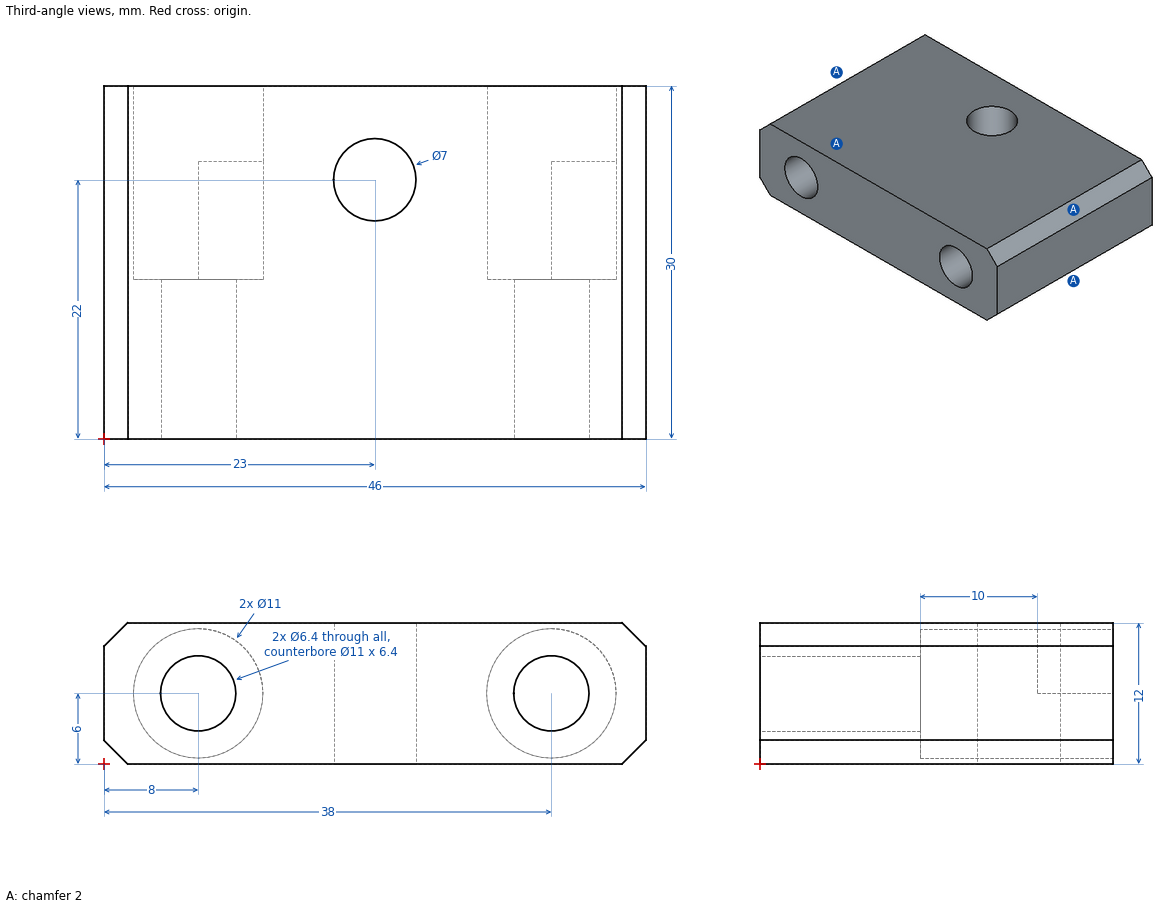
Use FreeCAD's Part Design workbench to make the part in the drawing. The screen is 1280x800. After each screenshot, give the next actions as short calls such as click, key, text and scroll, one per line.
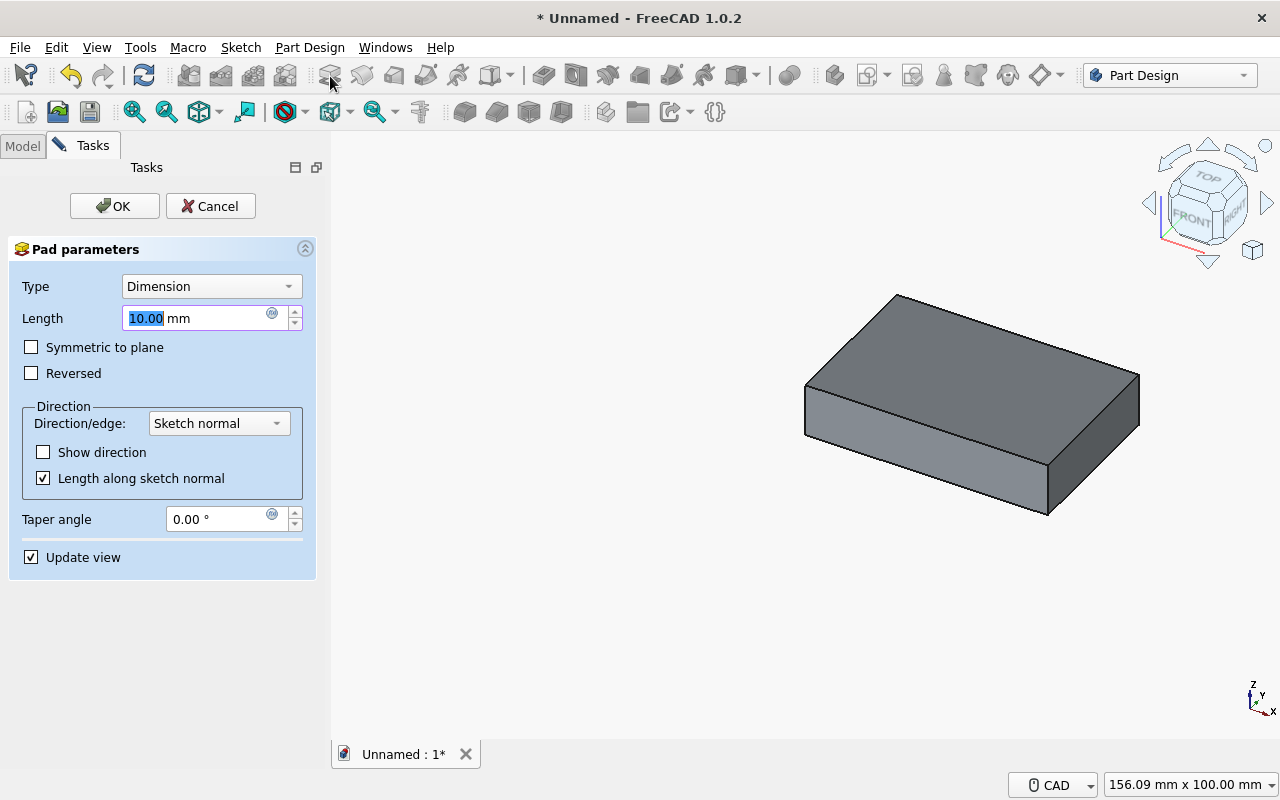
text(12)
key(Tab)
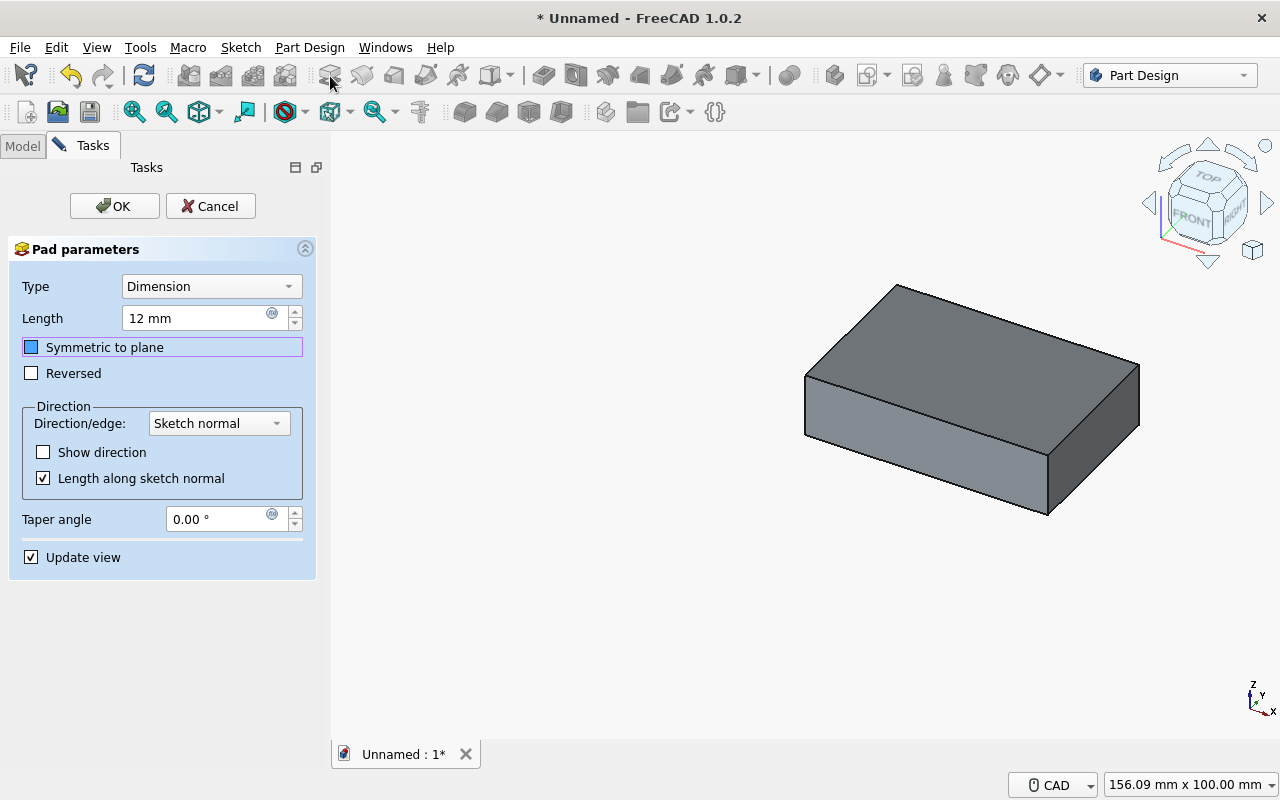
click(115, 206)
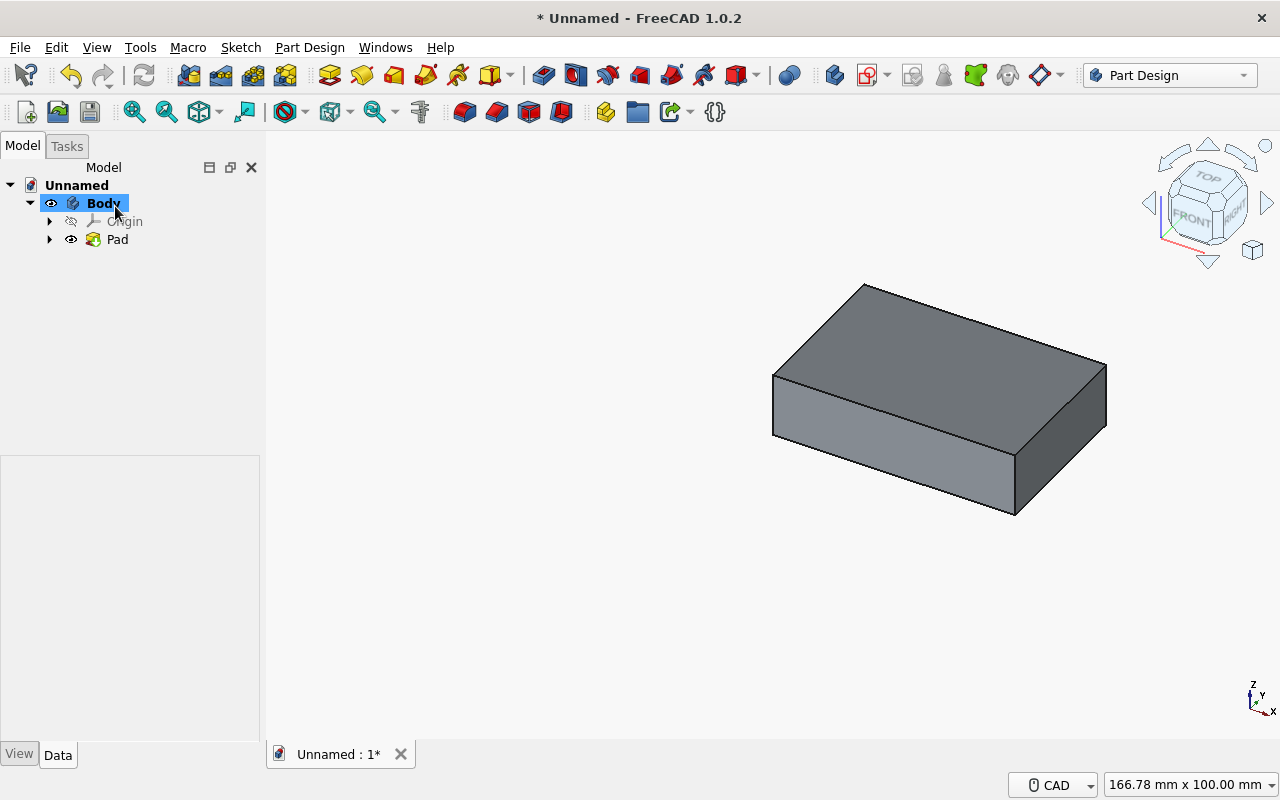
click(136, 112)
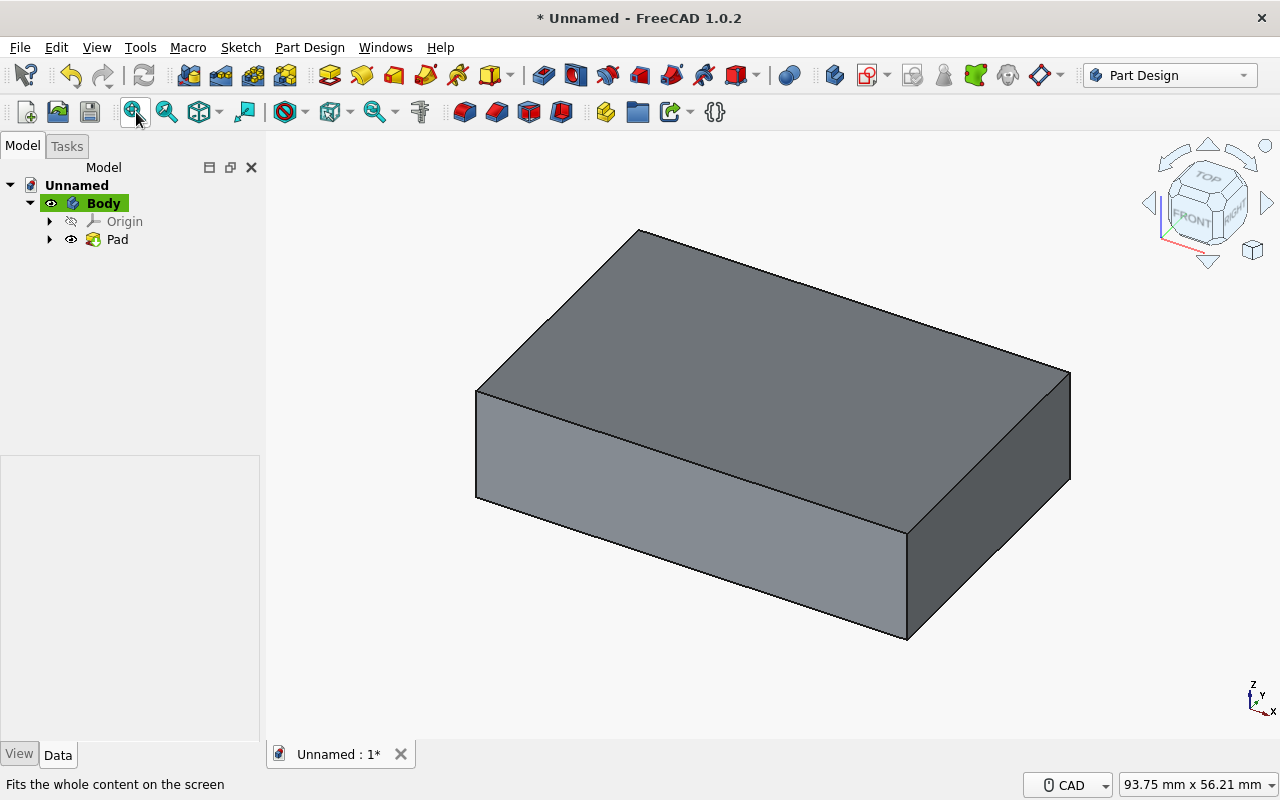
click(835, 401)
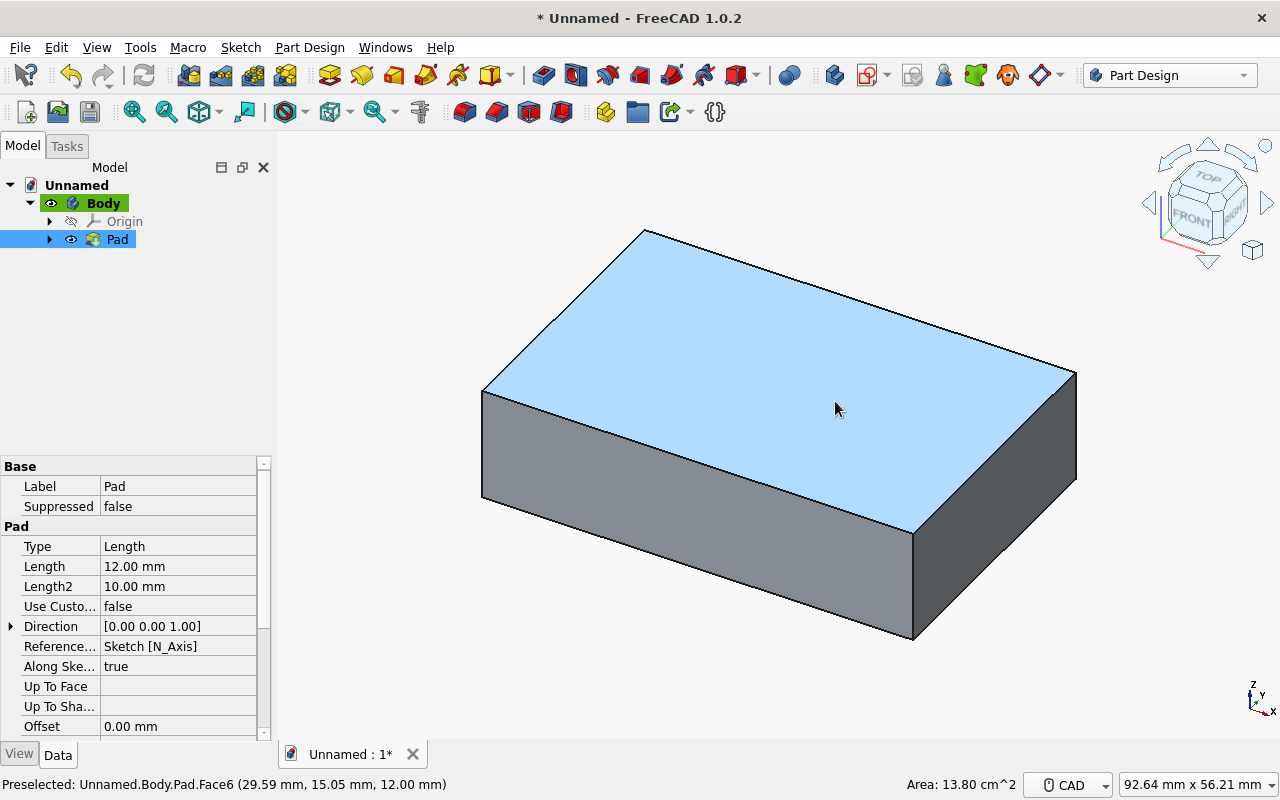
click(868, 76)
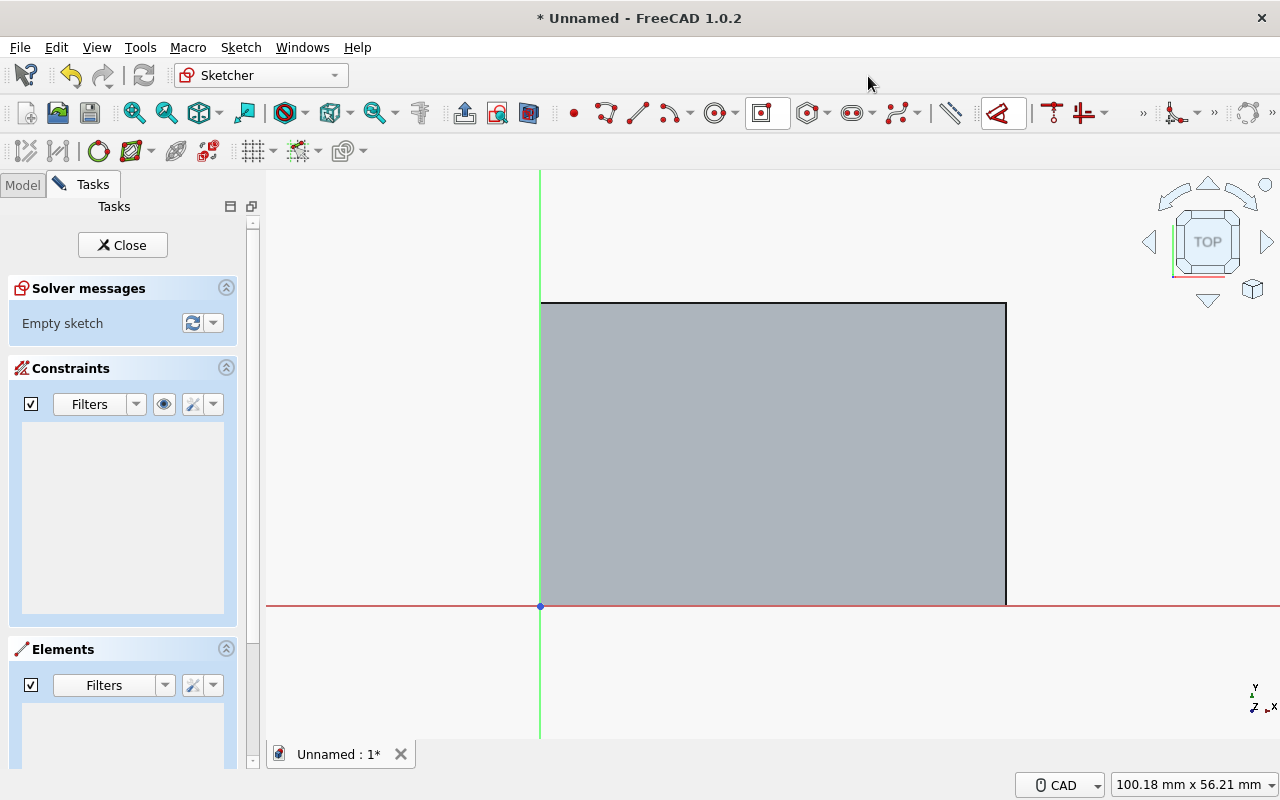
scroll(790, 366, up, 8)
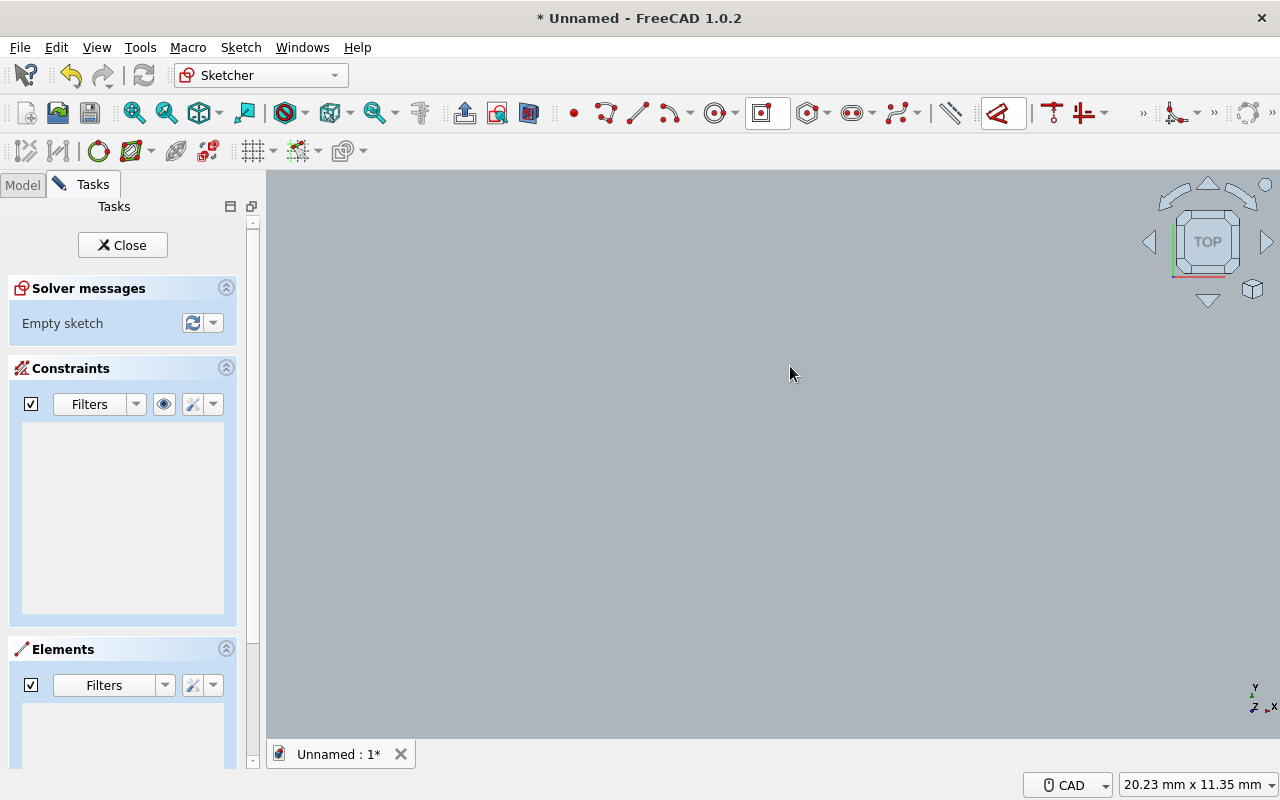
key(g)
key(c)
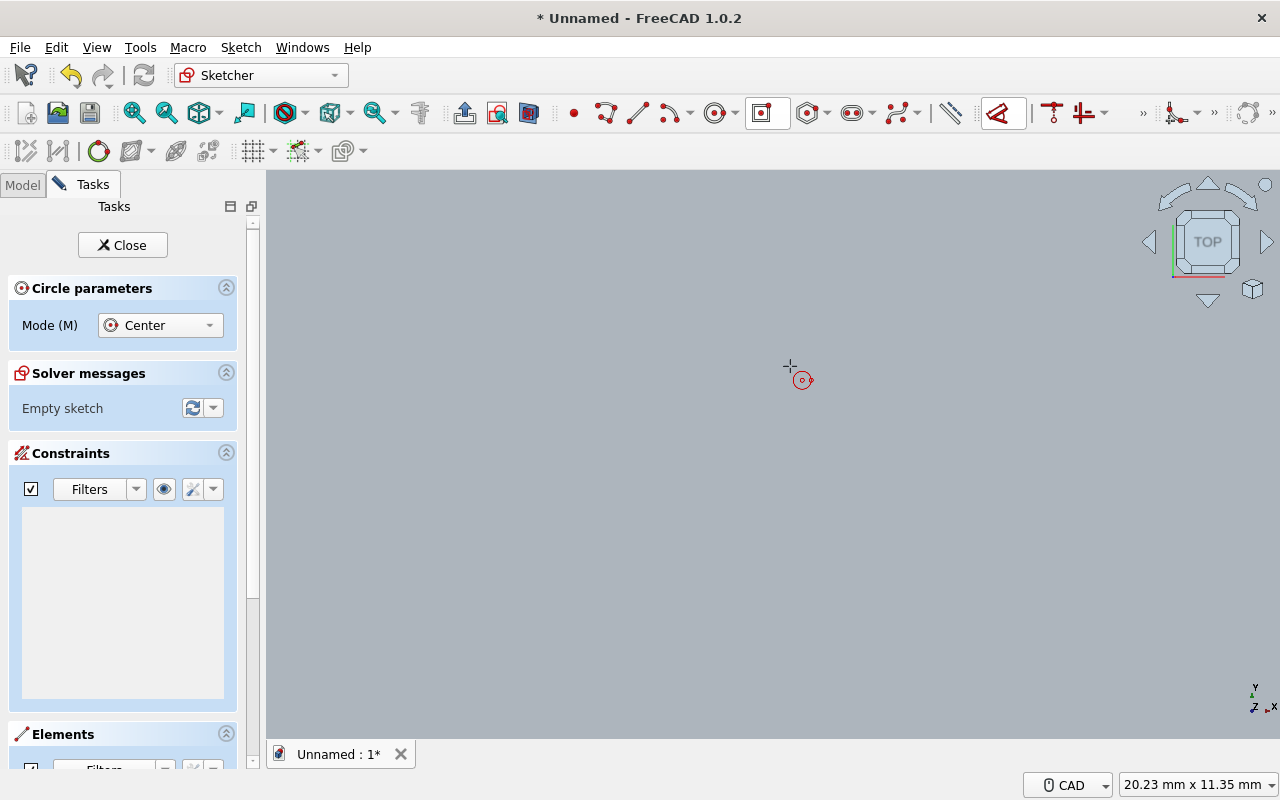
click(704, 452)
move(828, 328)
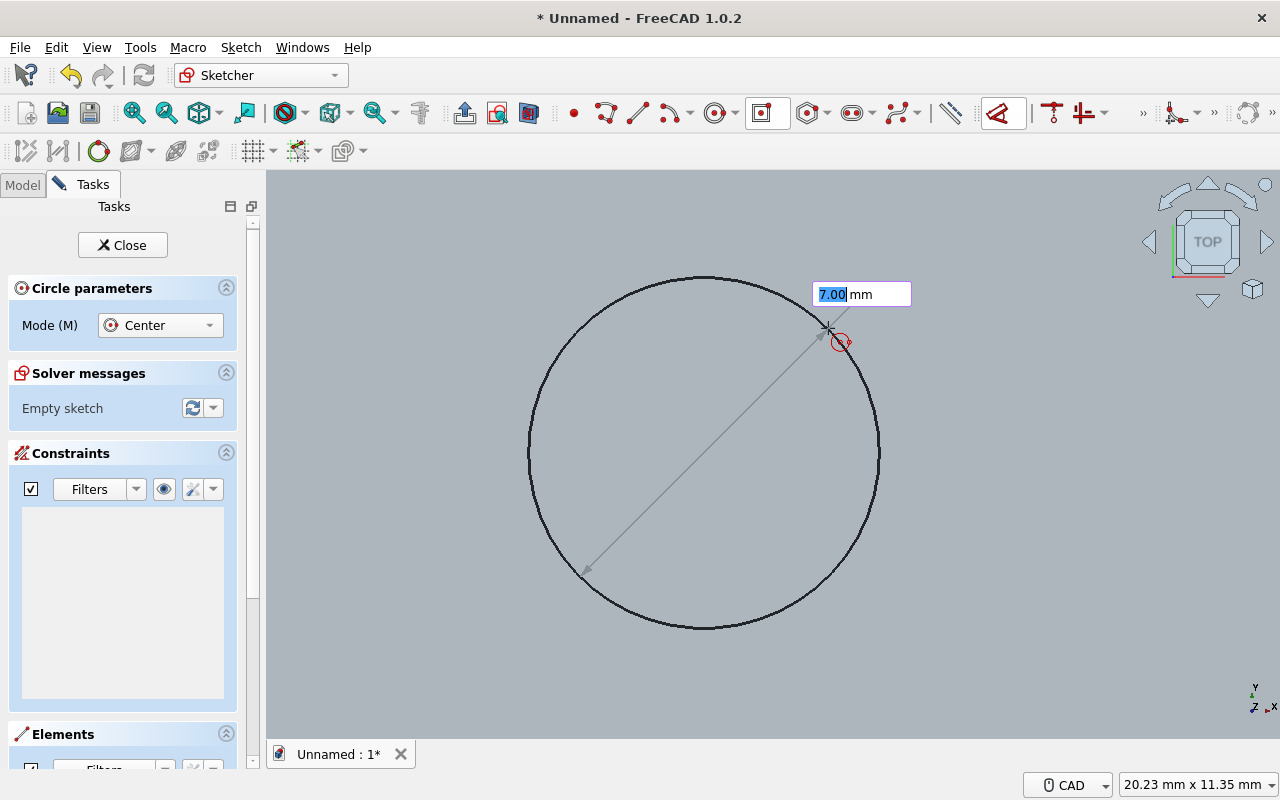
text(7)
key(Return)
key(Escape)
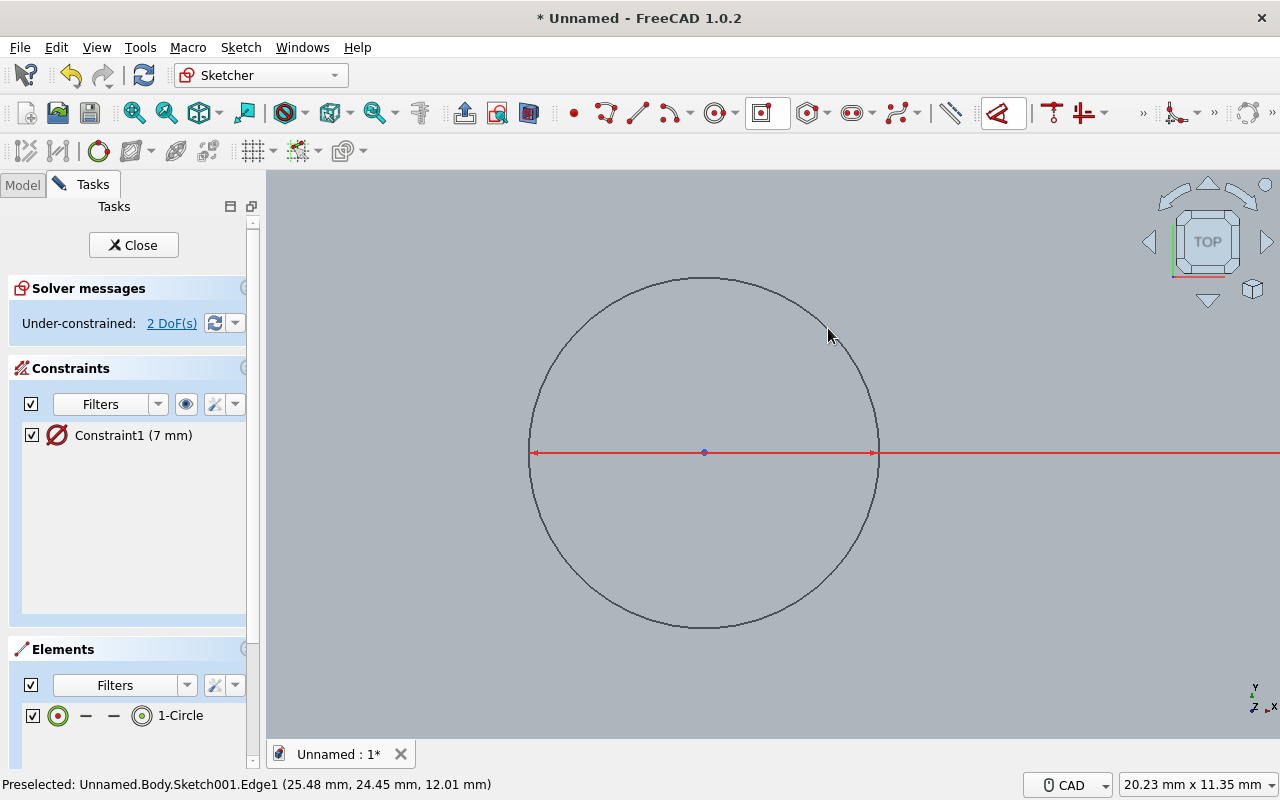
click(704, 453)